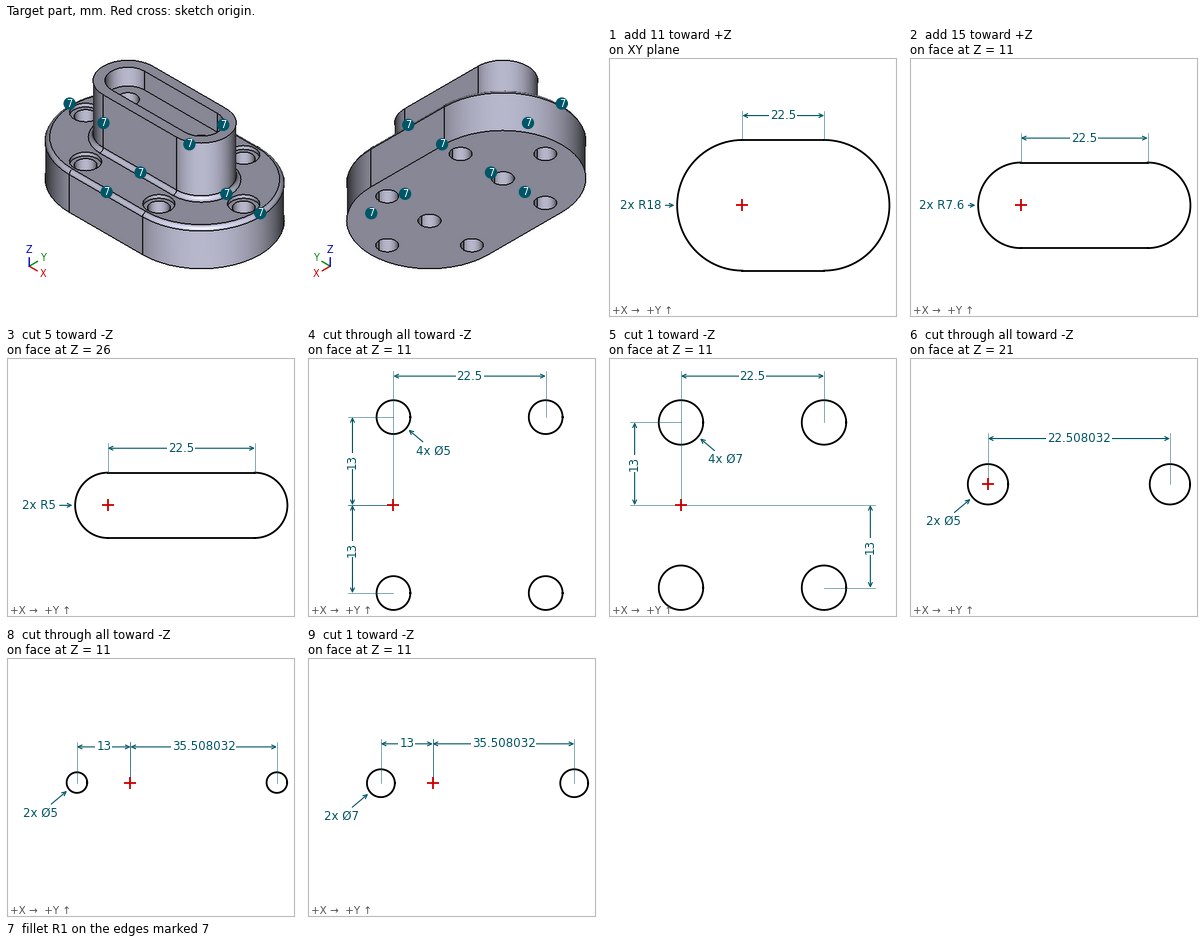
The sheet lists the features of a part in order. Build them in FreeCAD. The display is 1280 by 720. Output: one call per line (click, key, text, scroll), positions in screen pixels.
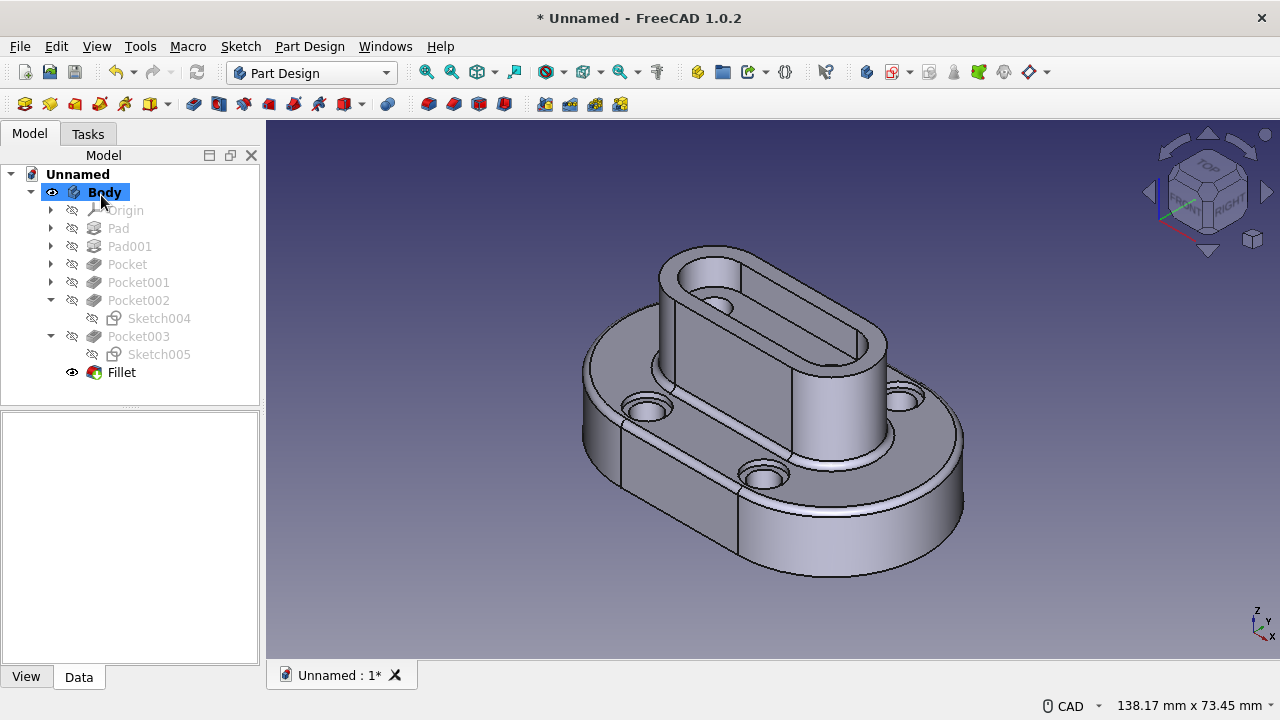
click(899, 473)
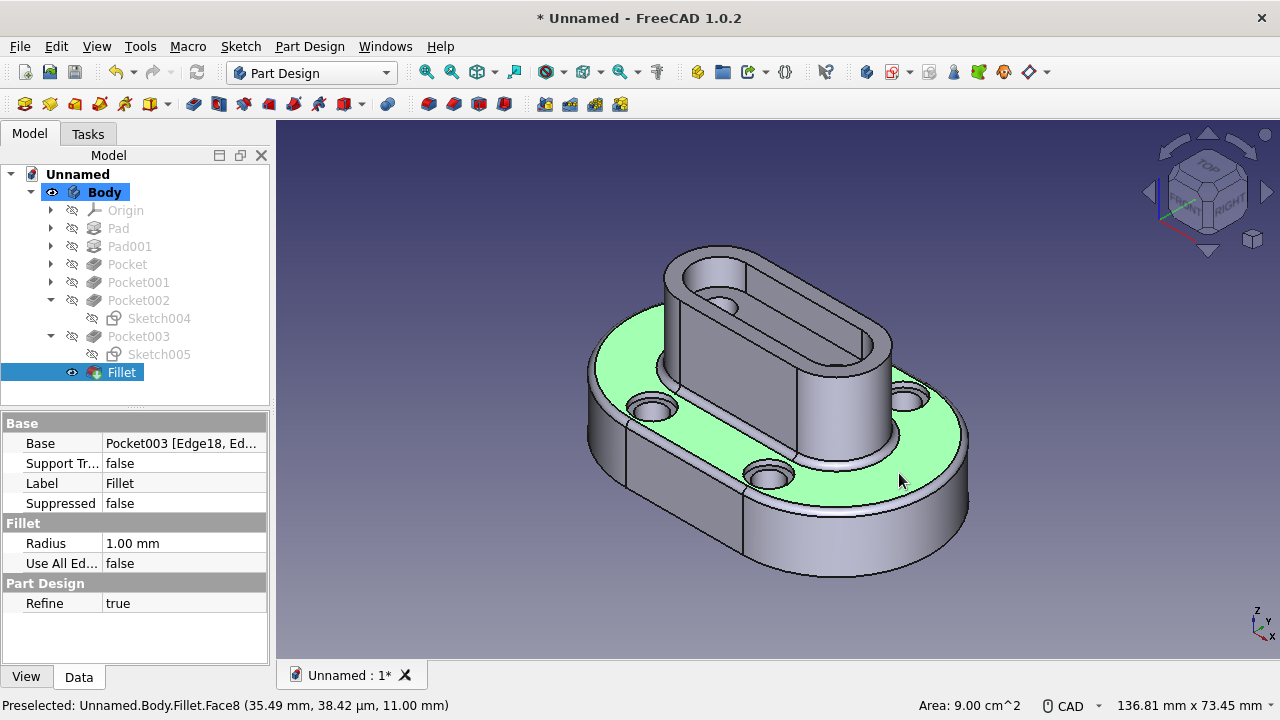
click(892, 72)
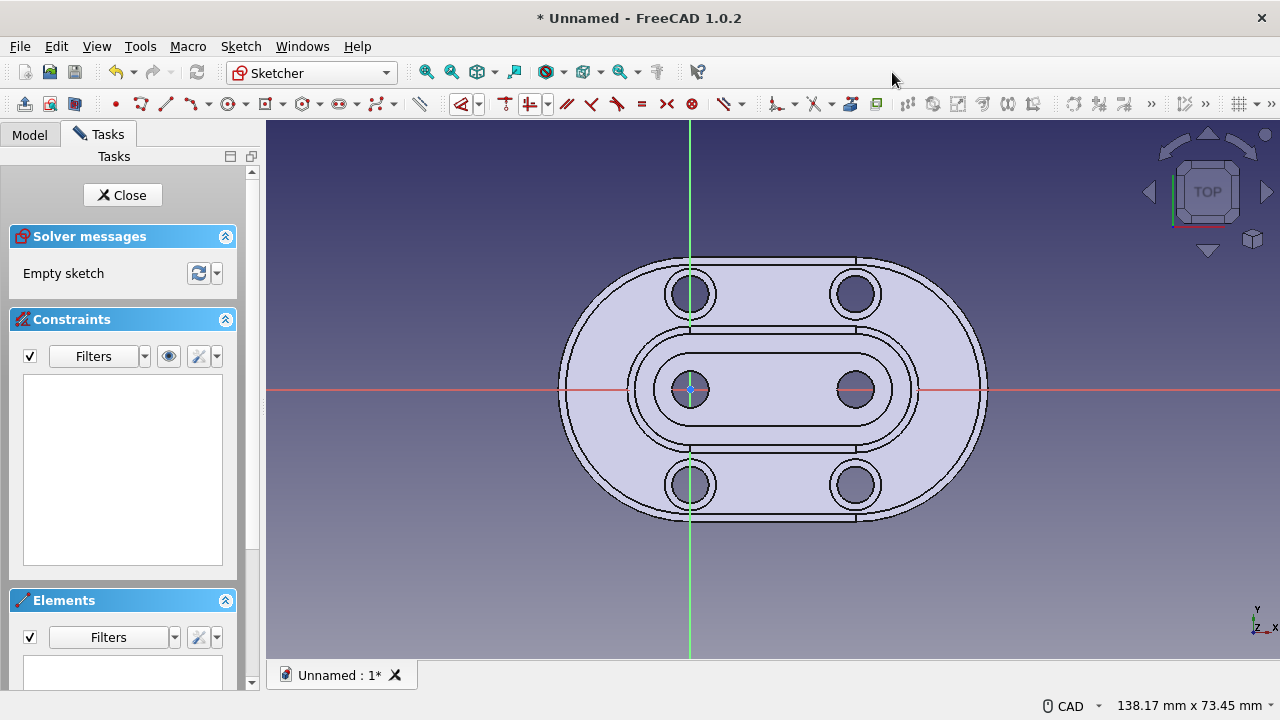
scroll(912, 390, up, 2)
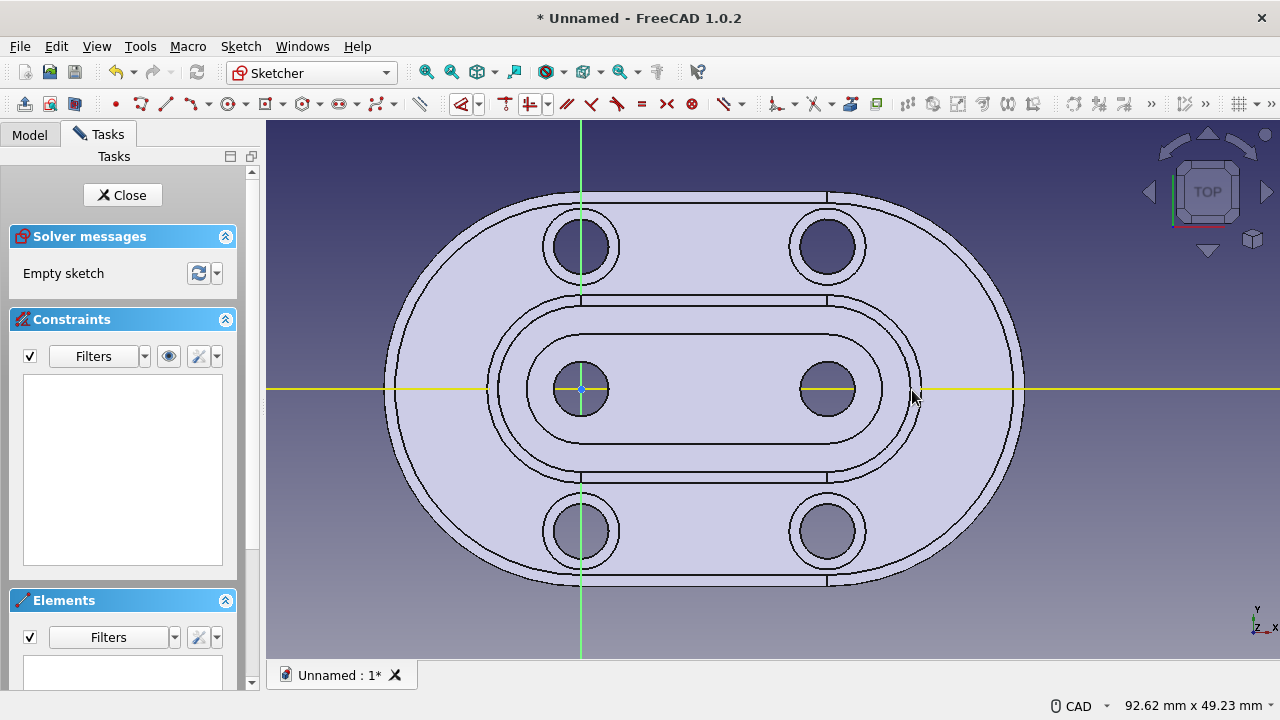
click(228, 104)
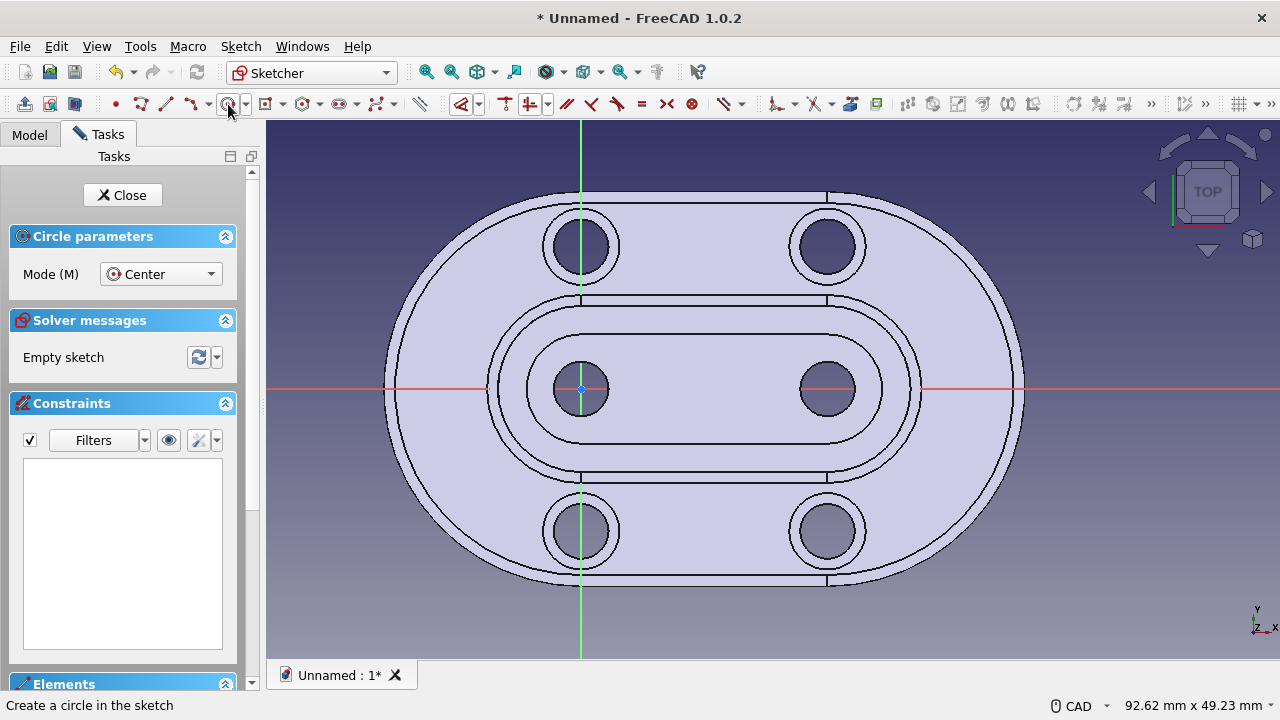
click(439, 389)
move(458, 370)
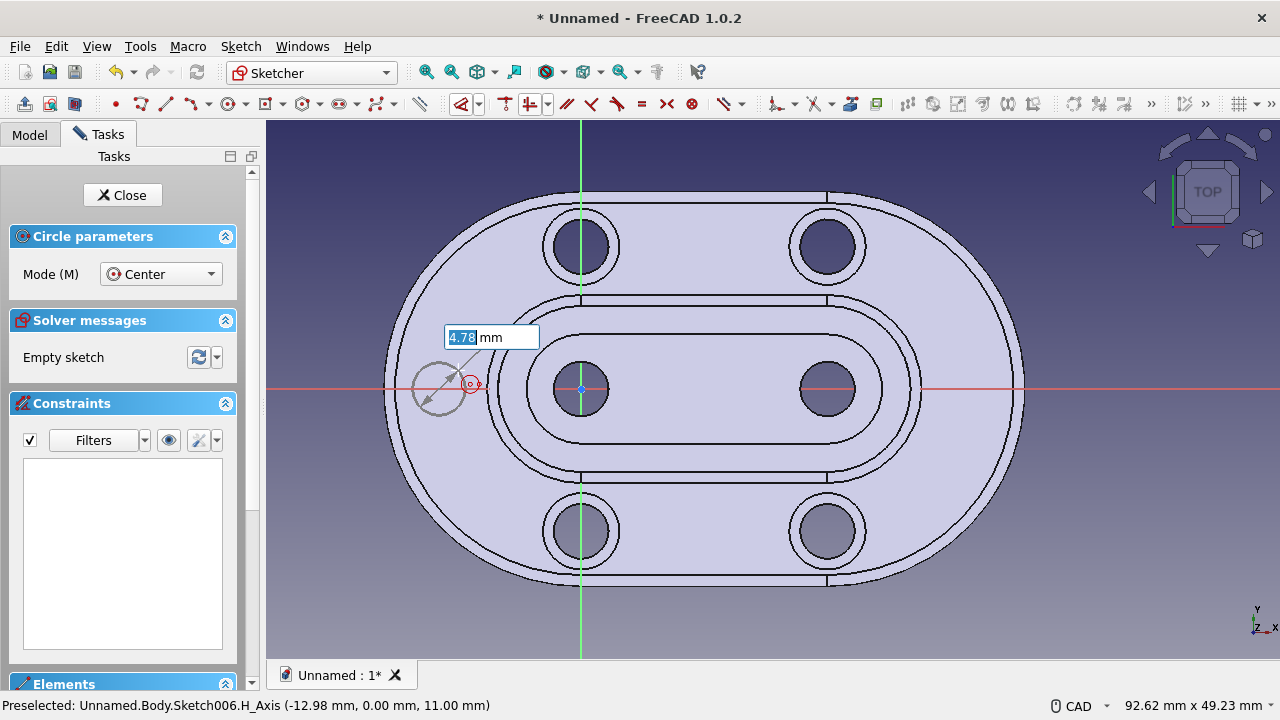
text(5)
key(Return)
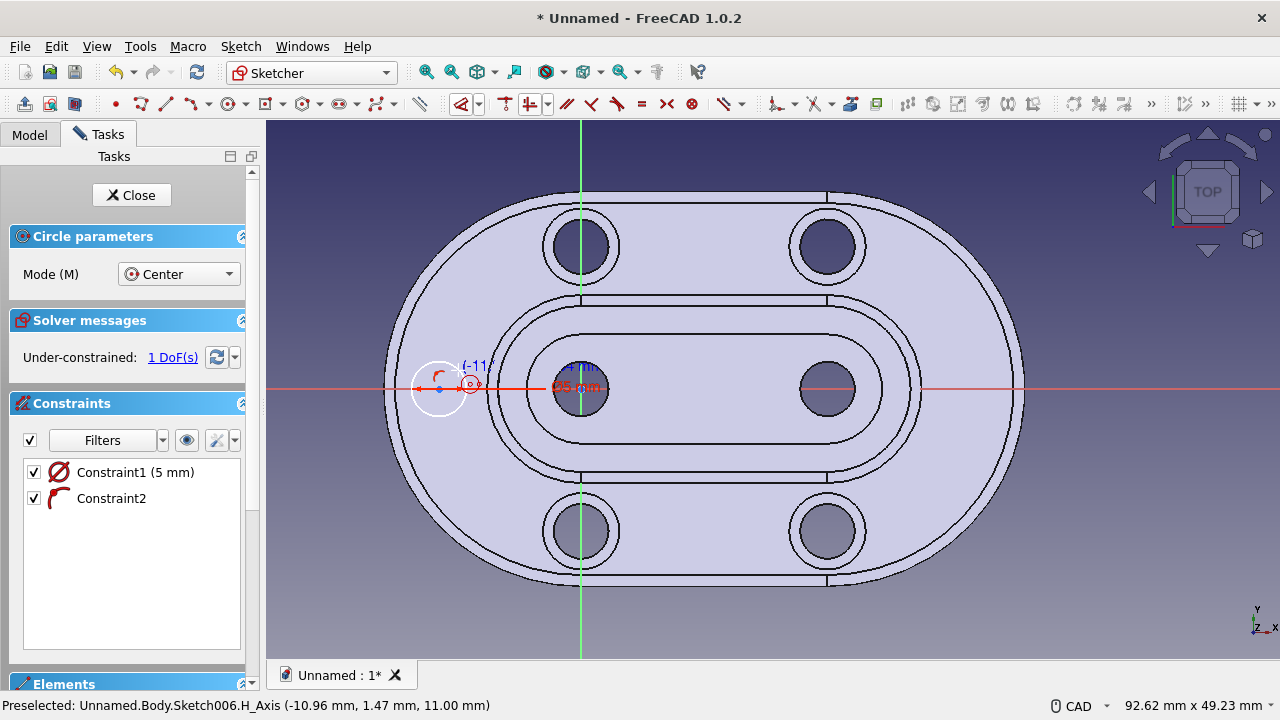
click(970, 389)
move(989, 370)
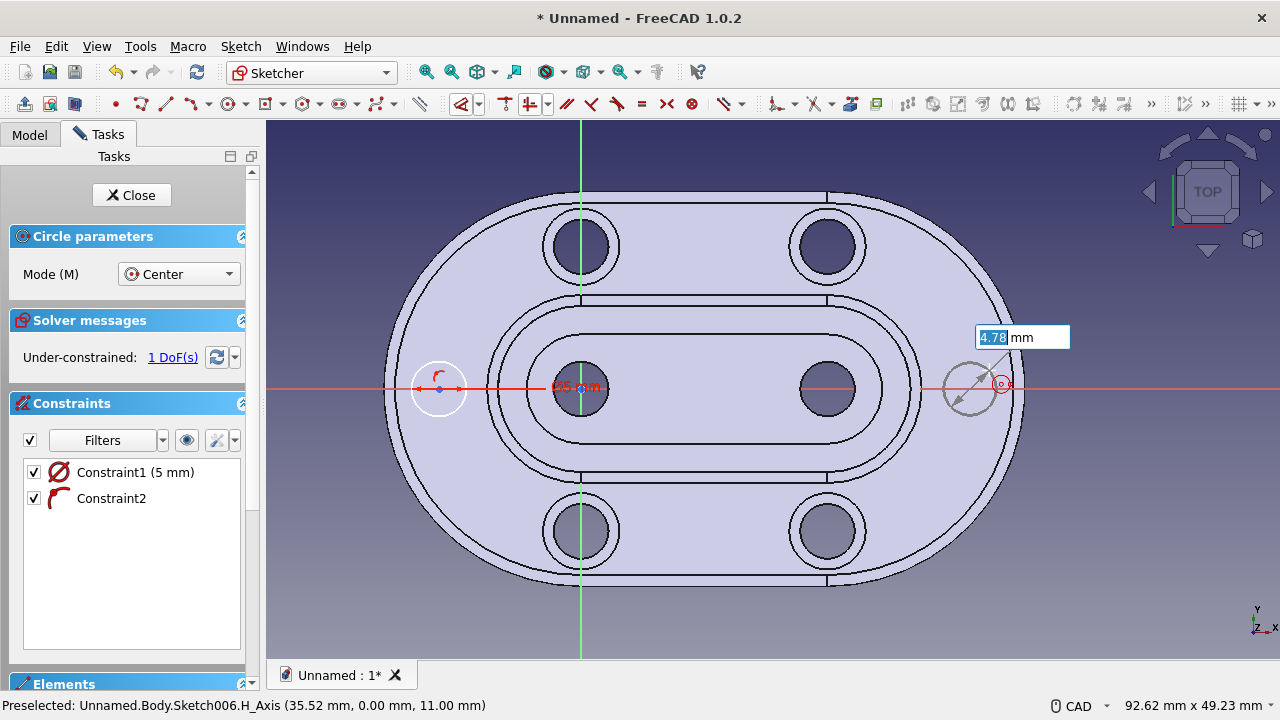
text(5)
key(Return)
key(Escape)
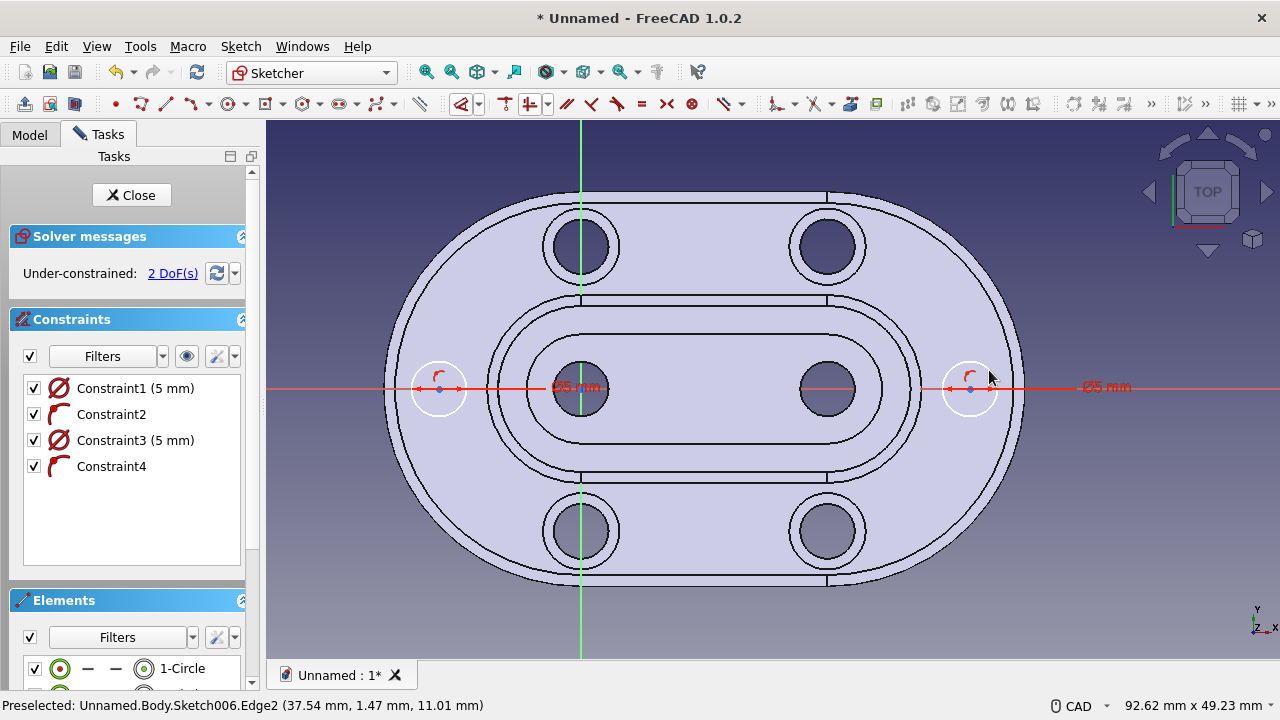
click(439, 389)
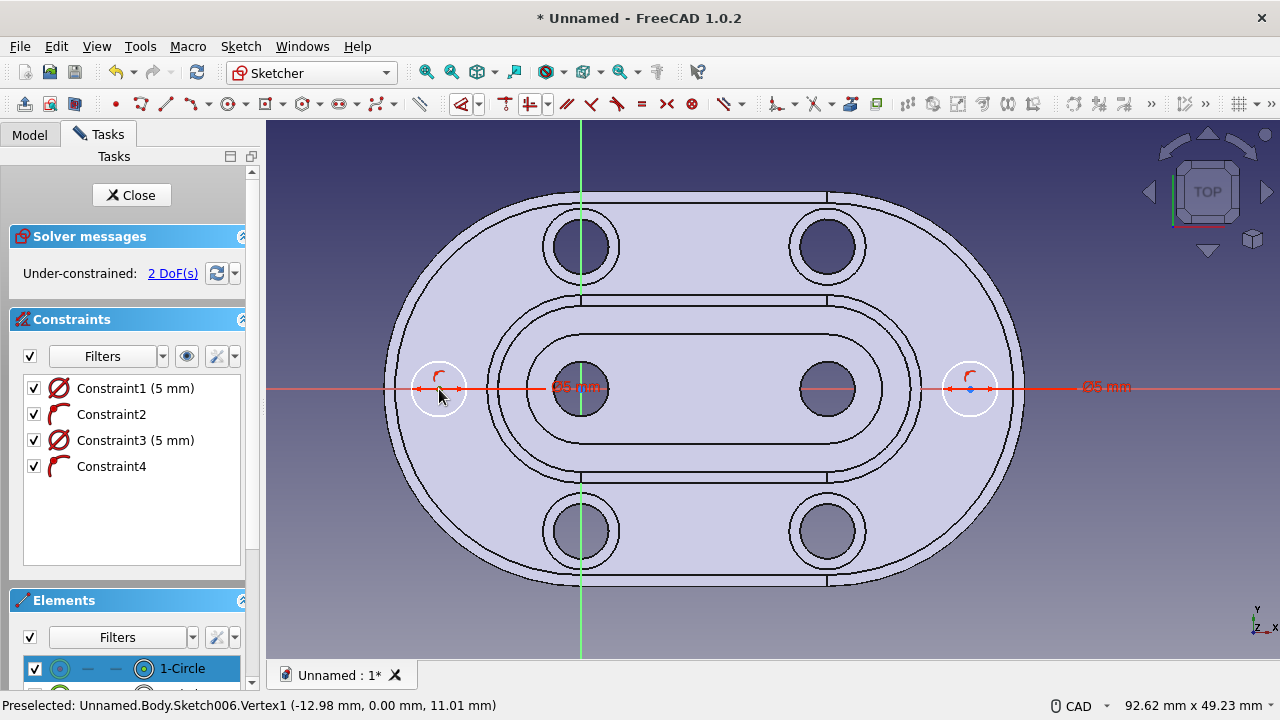
key(l)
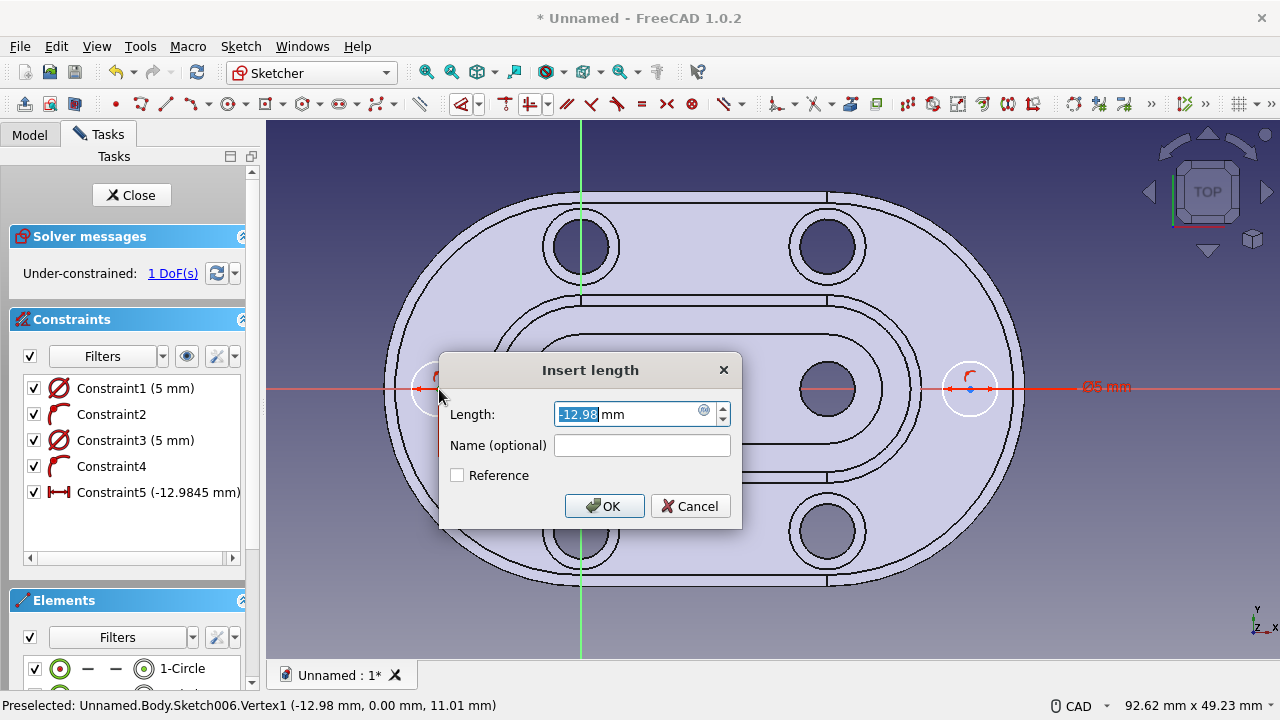
text(-13)
key(Return)